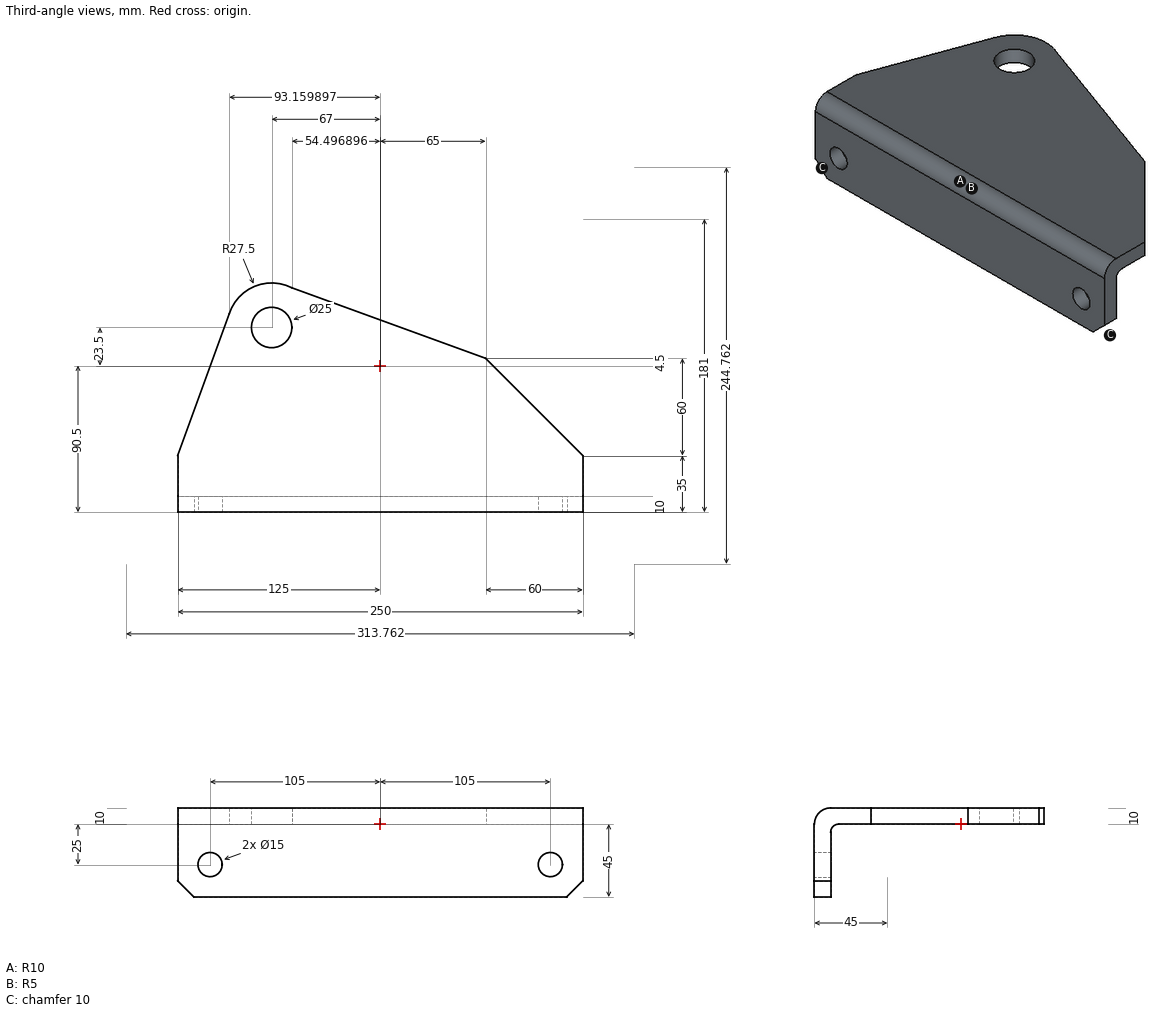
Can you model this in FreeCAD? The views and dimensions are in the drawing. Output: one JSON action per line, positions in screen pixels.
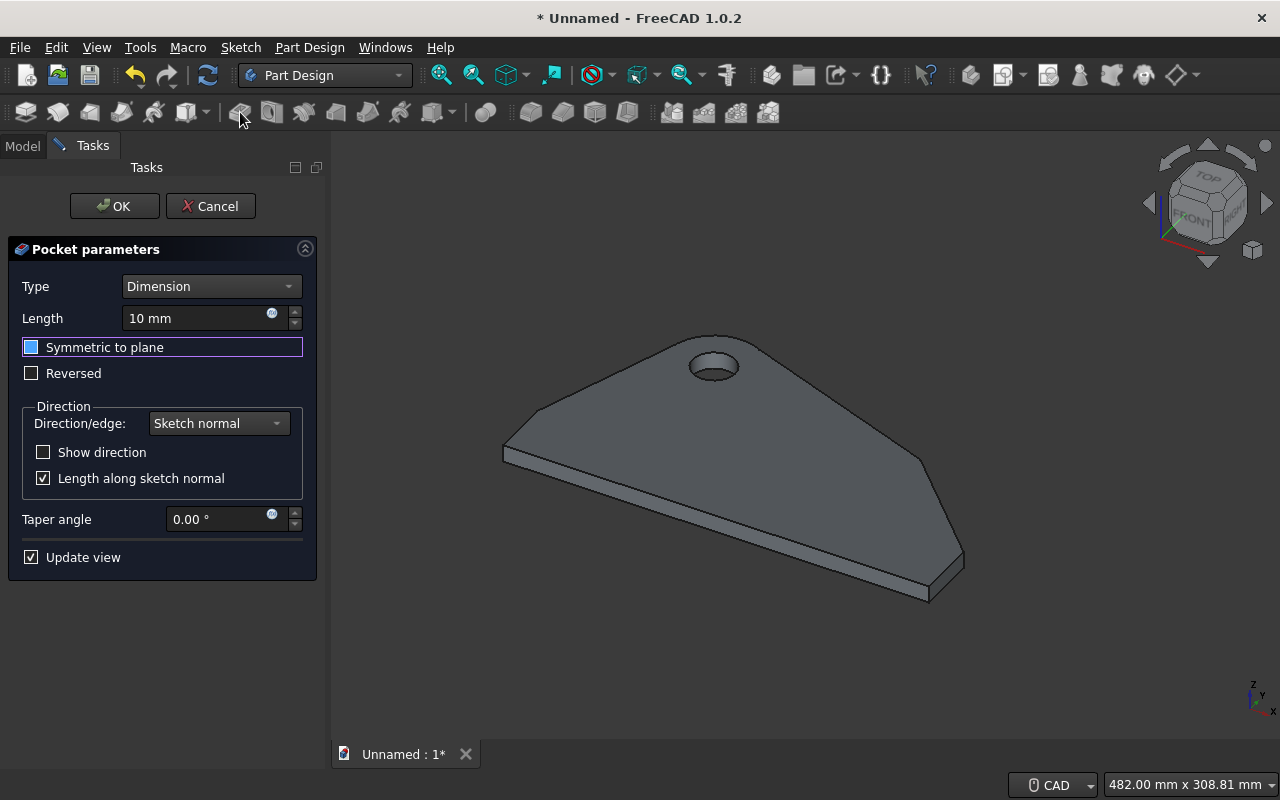
{"action": "left_click", "coordinate": [115, 206]}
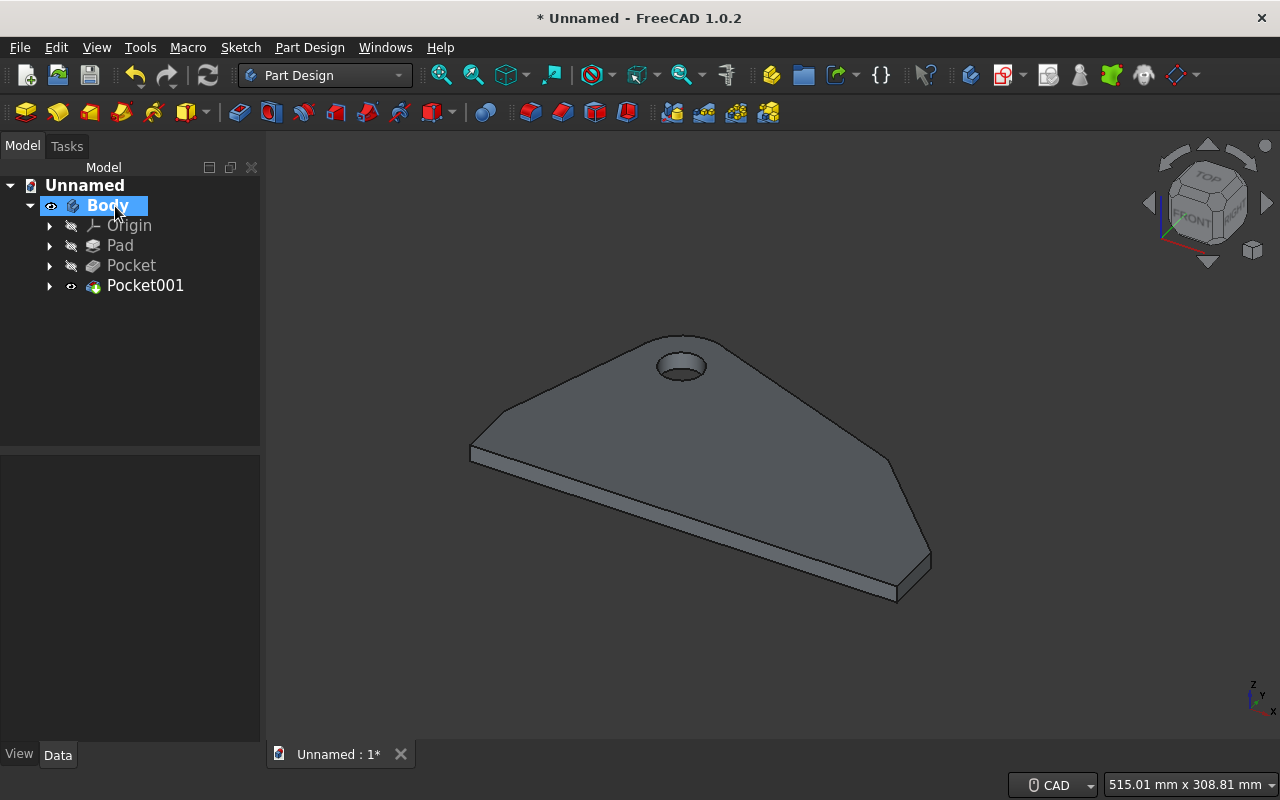
{"action": "key", "text": "5"}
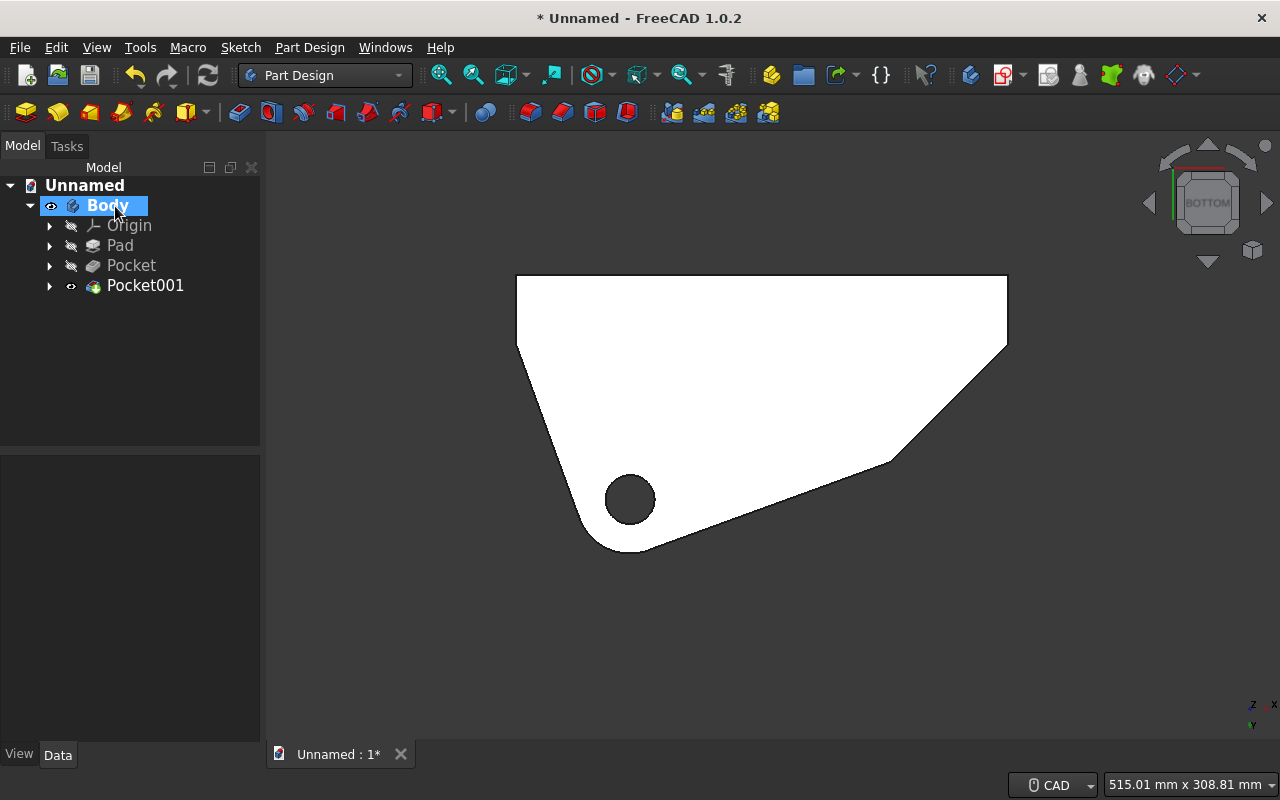
{"action": "left_click", "coordinate": [832, 374]}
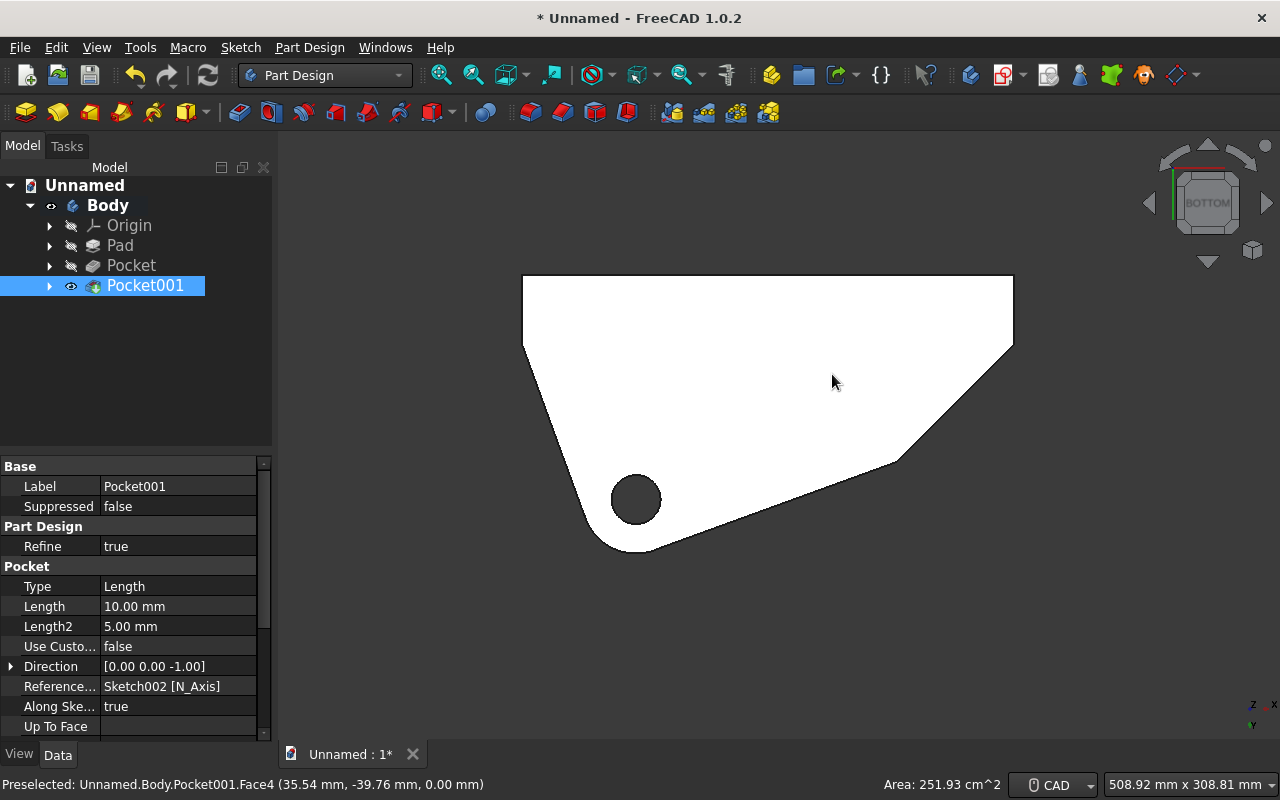
{"action": "left_click", "coordinate": [1004, 76]}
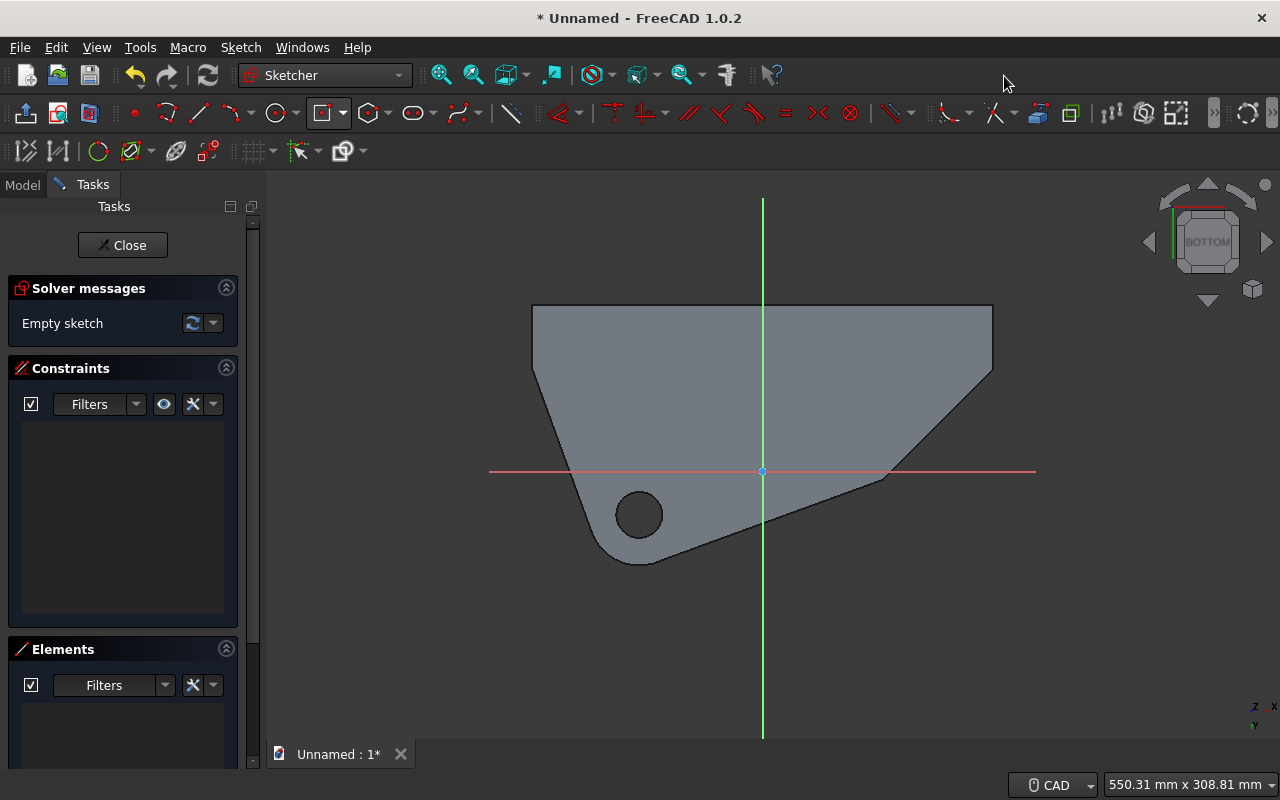
{"action": "left_click", "coordinate": [346, 114]}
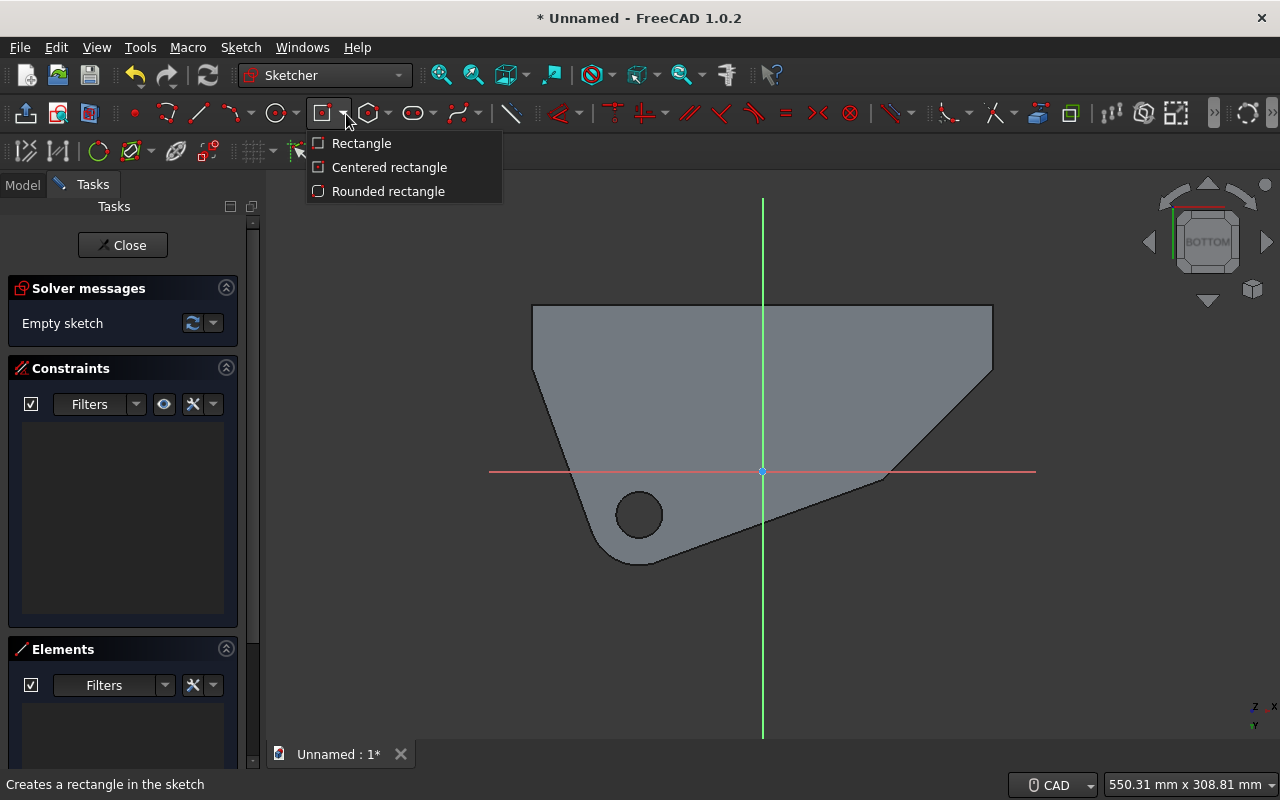
{"action": "left_click", "coordinate": [404, 143]}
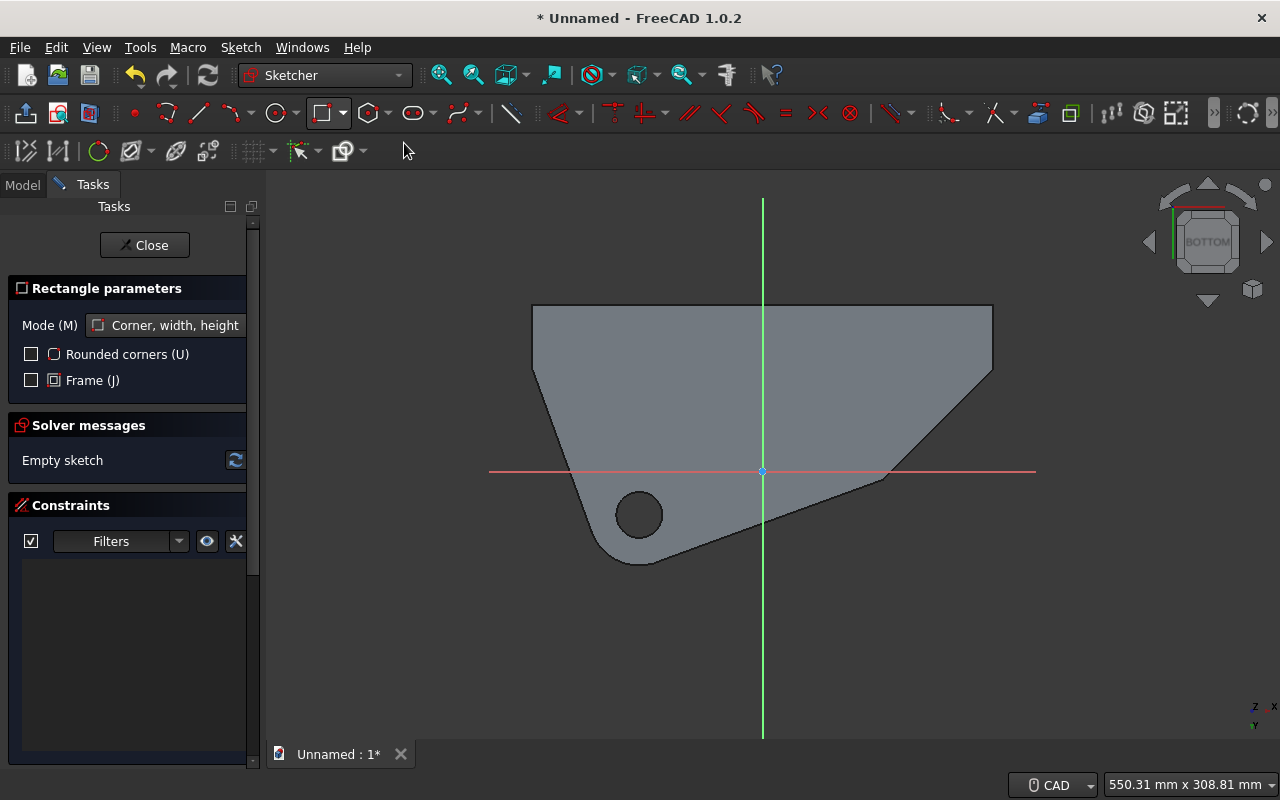
{"action": "left_click", "coordinate": [532, 305]}
{"action": "mouse_move", "coordinate": [993, 323]}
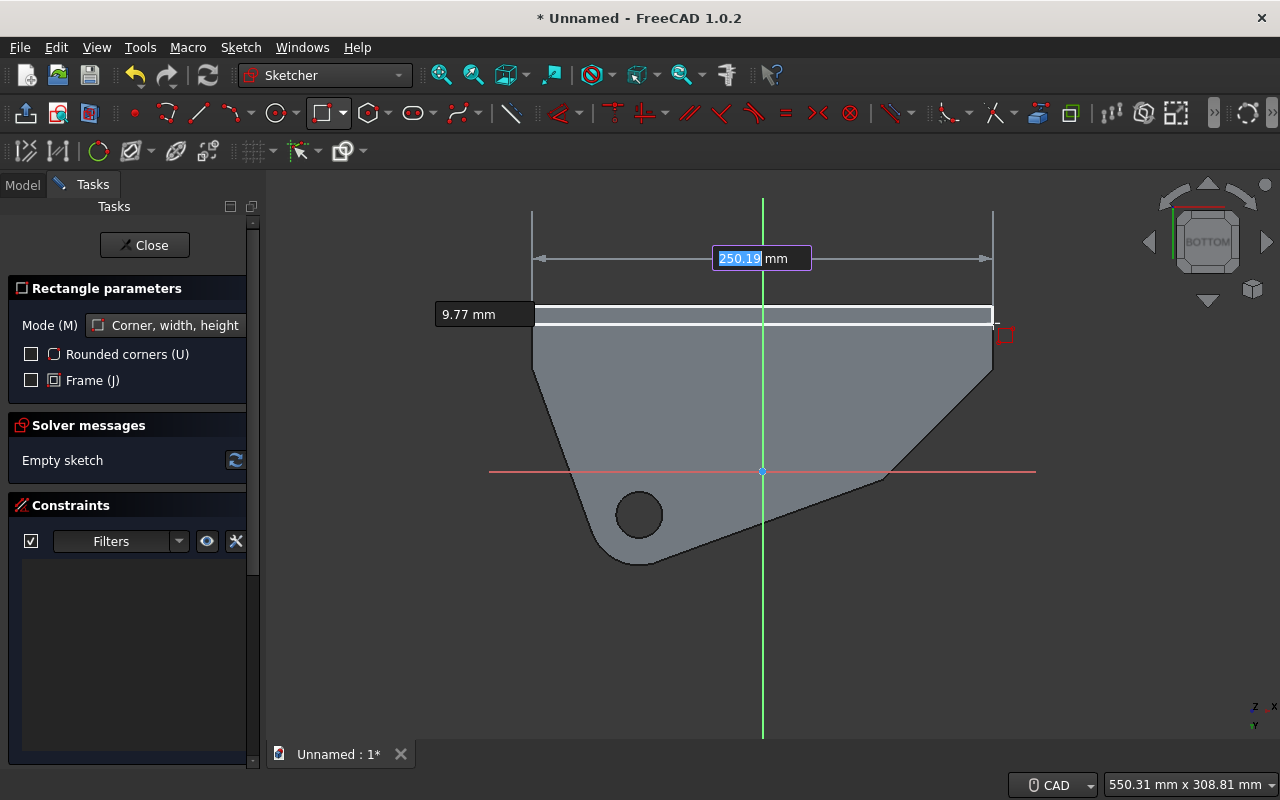
{"action": "type", "text": "250"}
{"action": "key", "text": "Tab"}
{"action": "type", "text": "10"}
{"action": "key", "text": "Return"}
{"action": "key", "text": "Escape"}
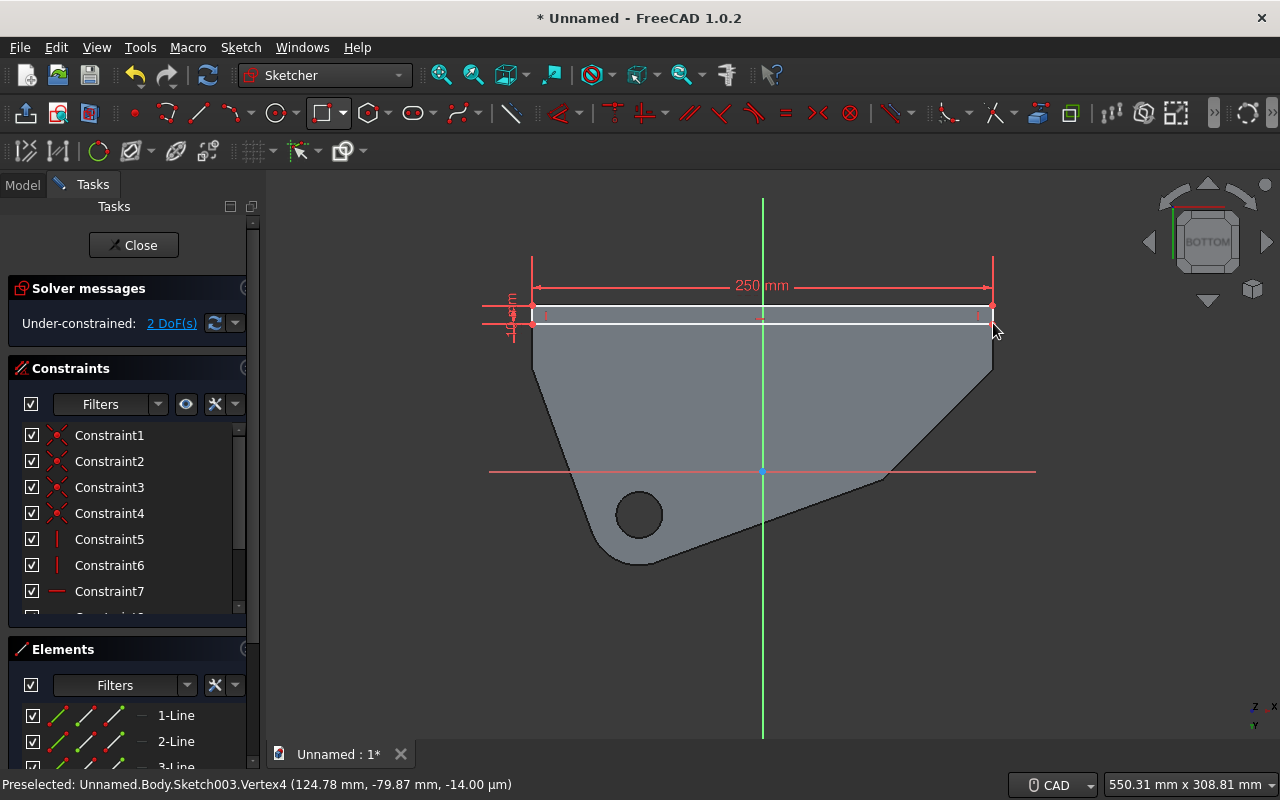
{"action": "key", "text": "d"}